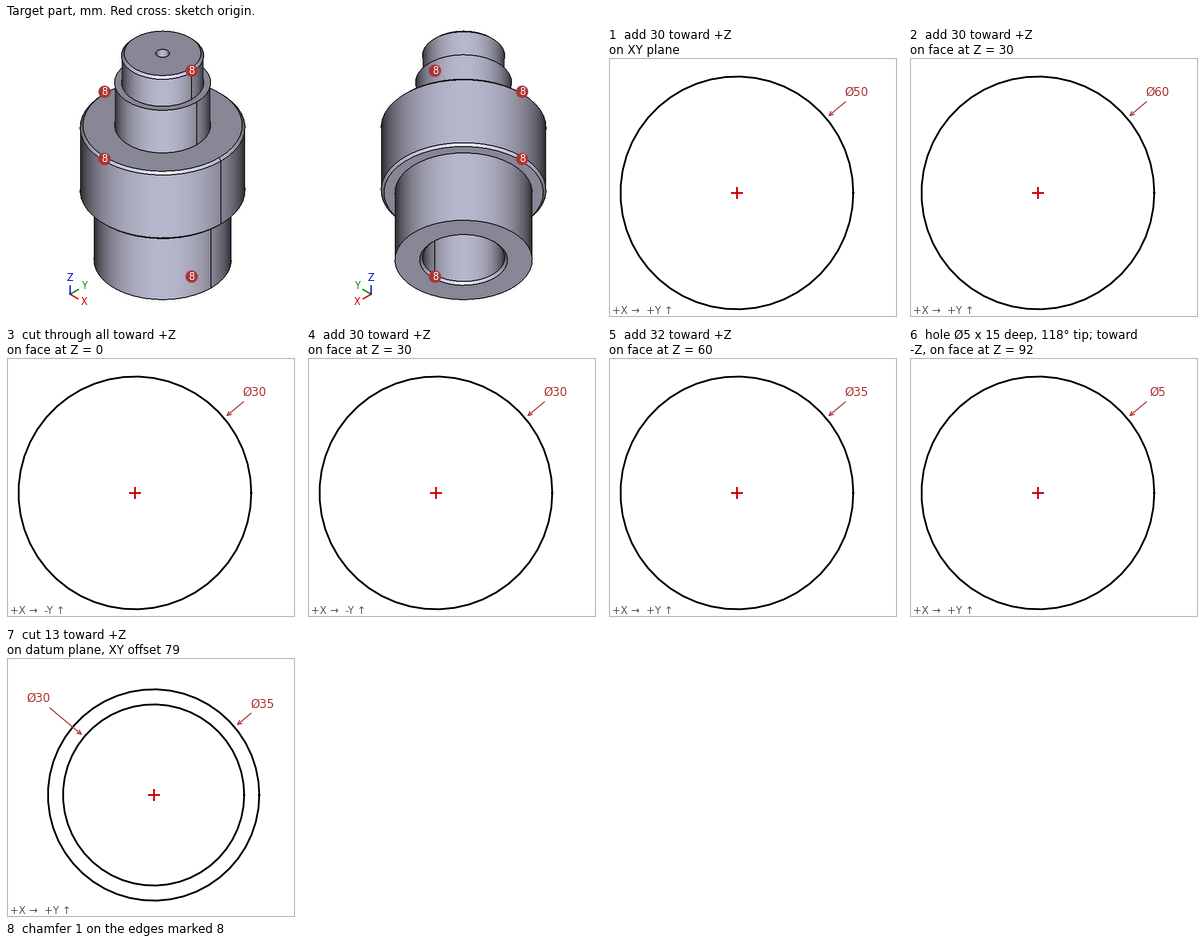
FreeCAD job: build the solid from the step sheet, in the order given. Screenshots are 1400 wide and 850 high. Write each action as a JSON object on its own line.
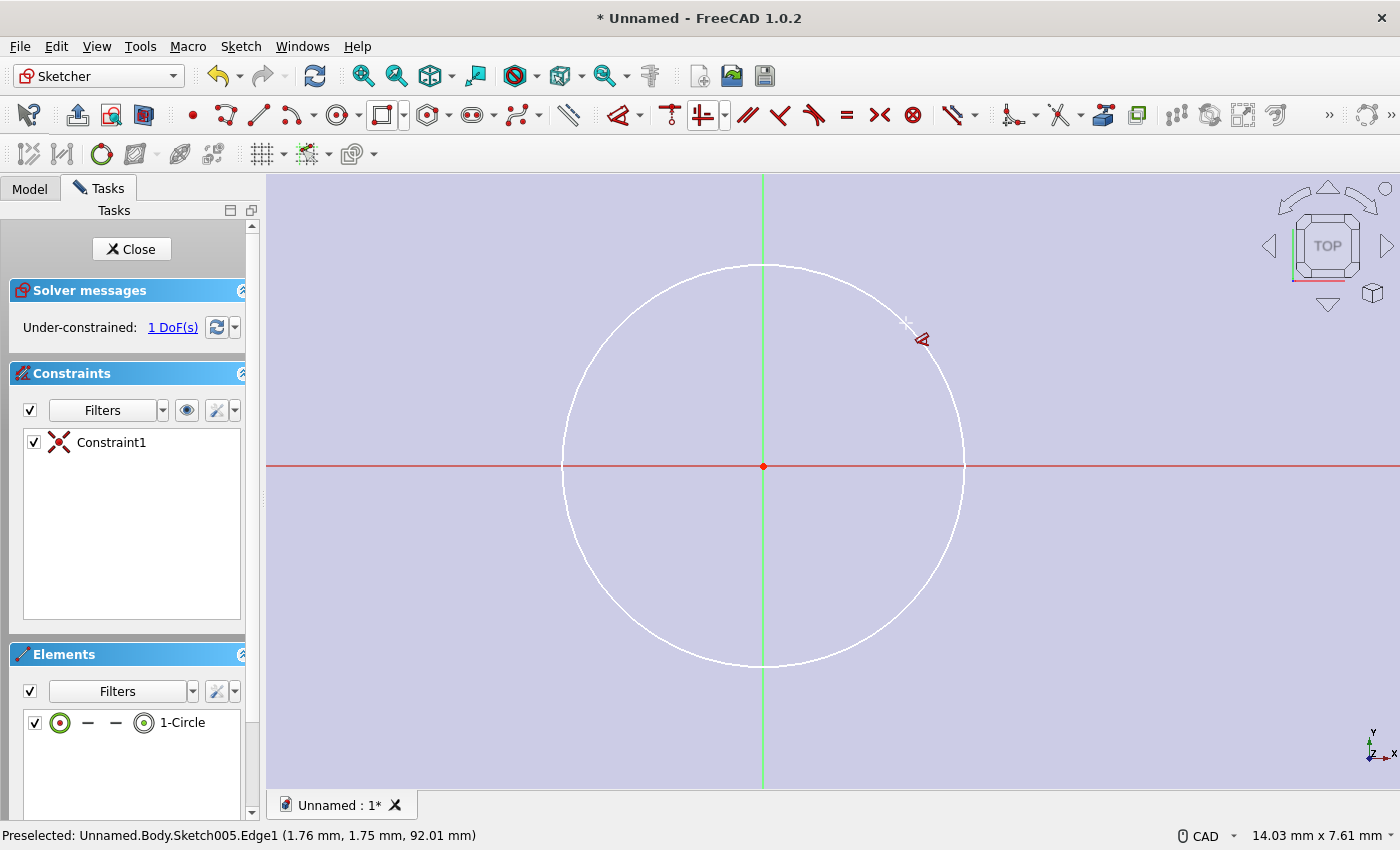
{"action": "left_click", "coordinate": [905, 323]}
{"action": "left_click", "coordinate": [928, 300]}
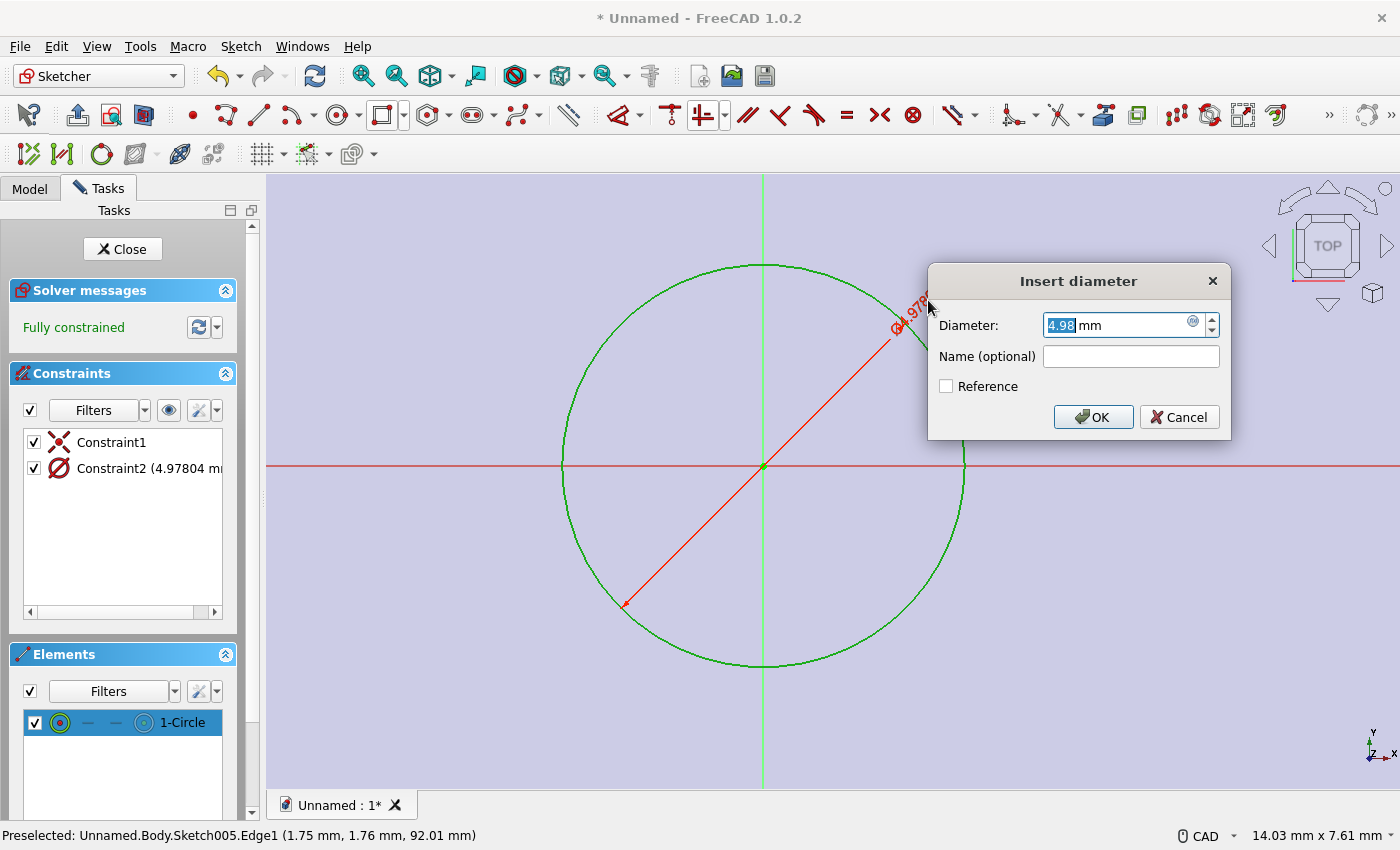
{"action": "type", "text": "5"}
{"action": "key", "text": "Return"}
{"action": "key", "text": "Escape"}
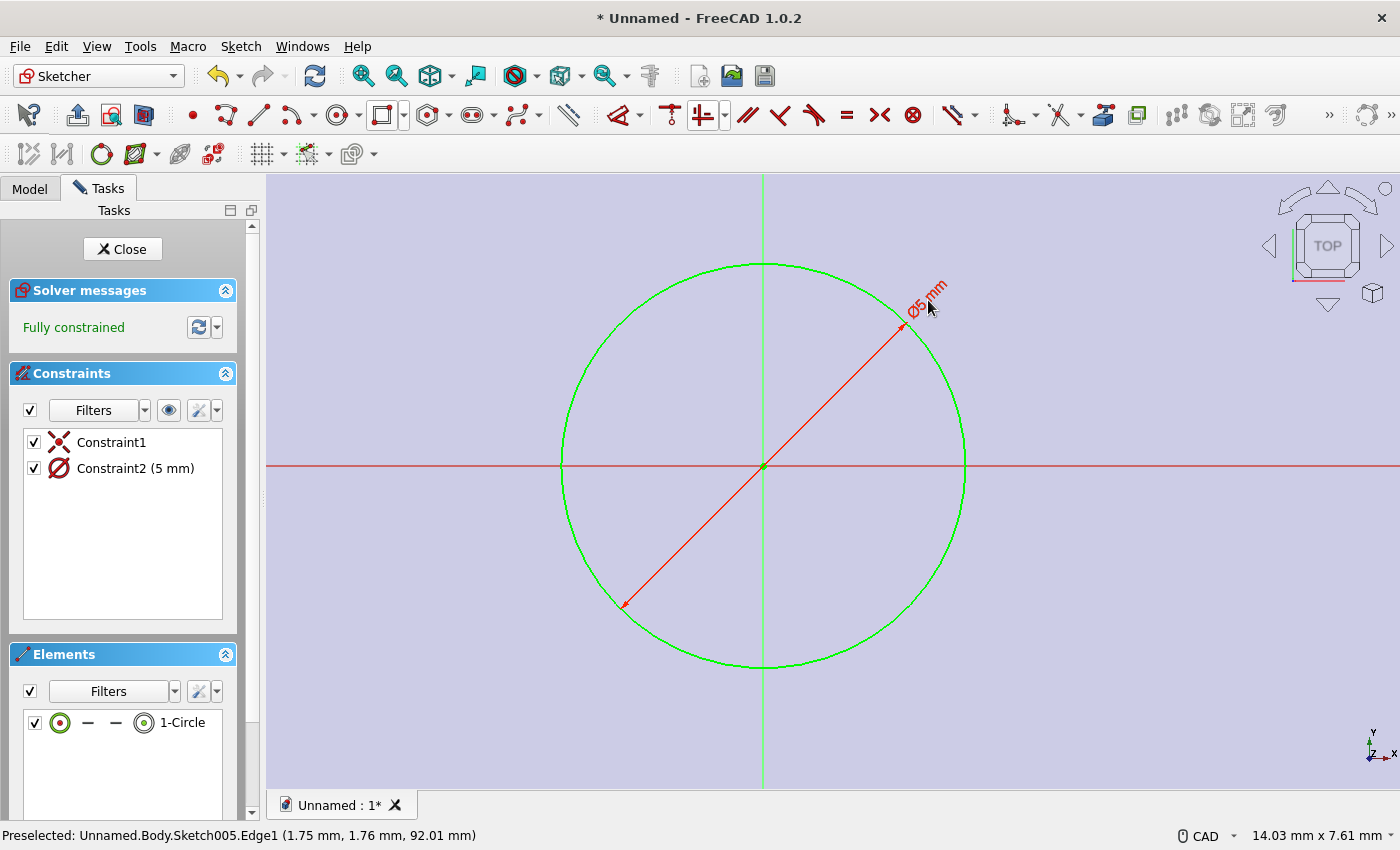
{"action": "left_click", "coordinate": [123, 249]}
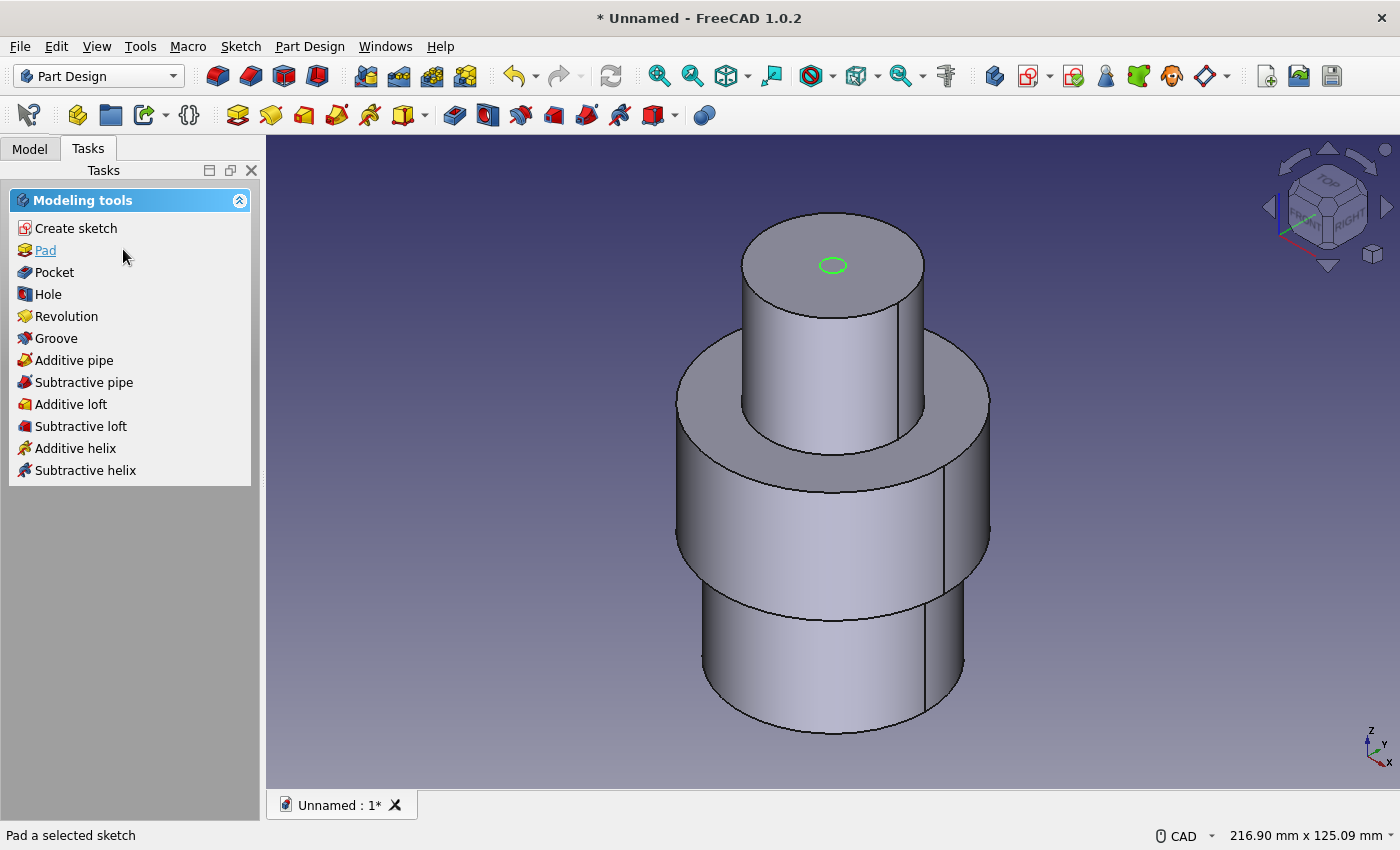
{"action": "left_click", "coordinate": [488, 116]}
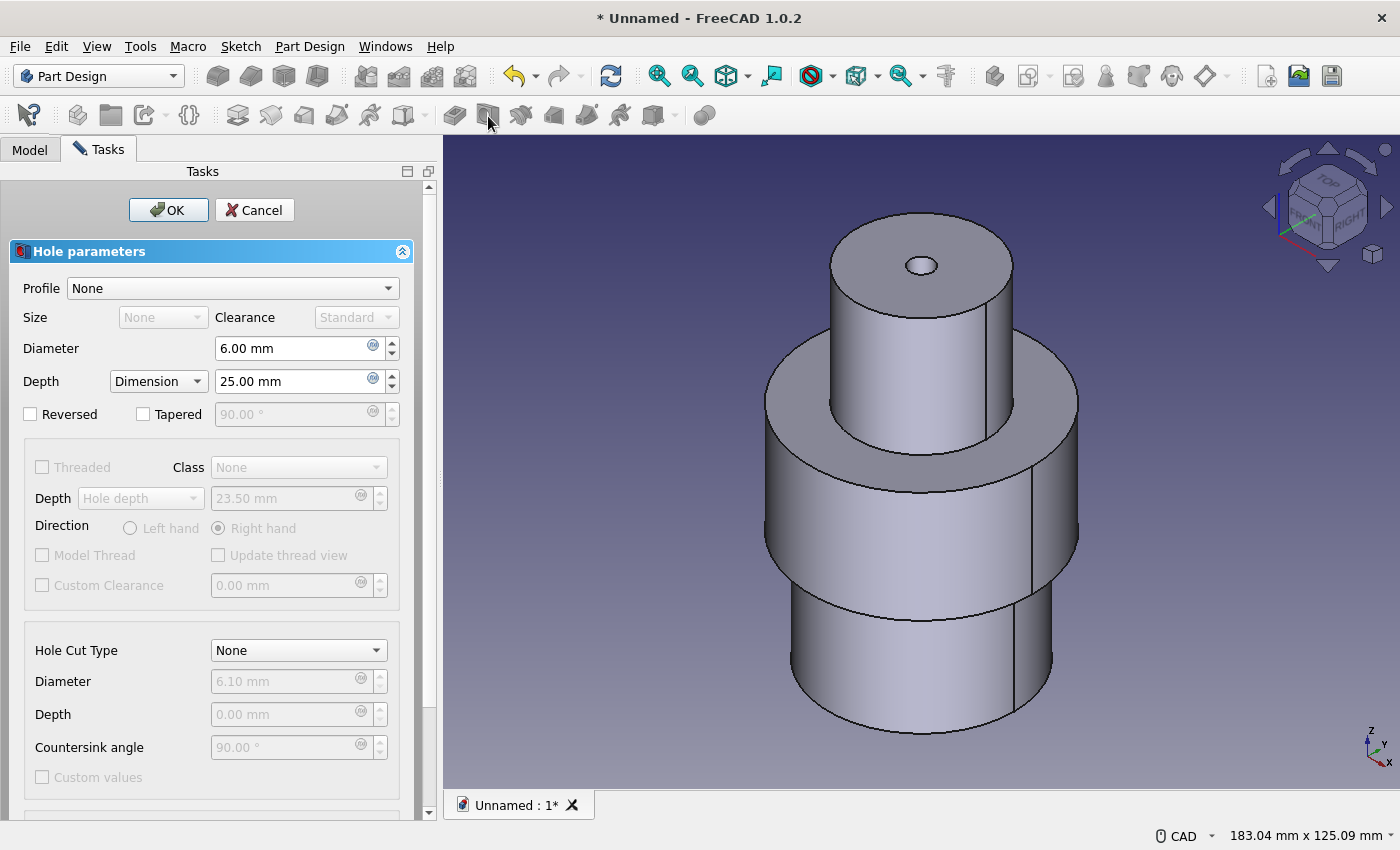
{"action": "triple_click", "coordinate": [300, 348]}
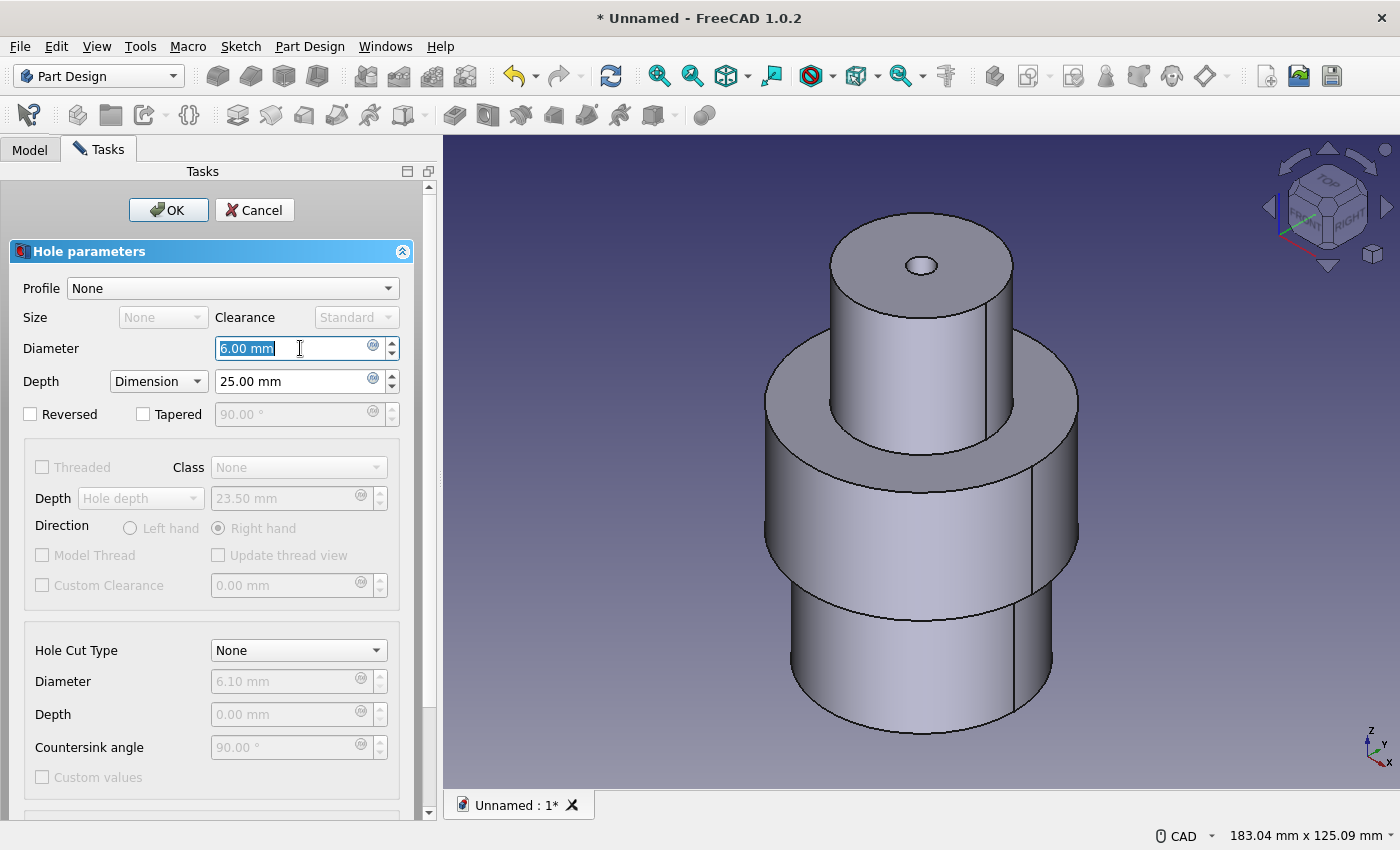
{"action": "type", "text": "5"}
{"action": "key", "text": "Tab"}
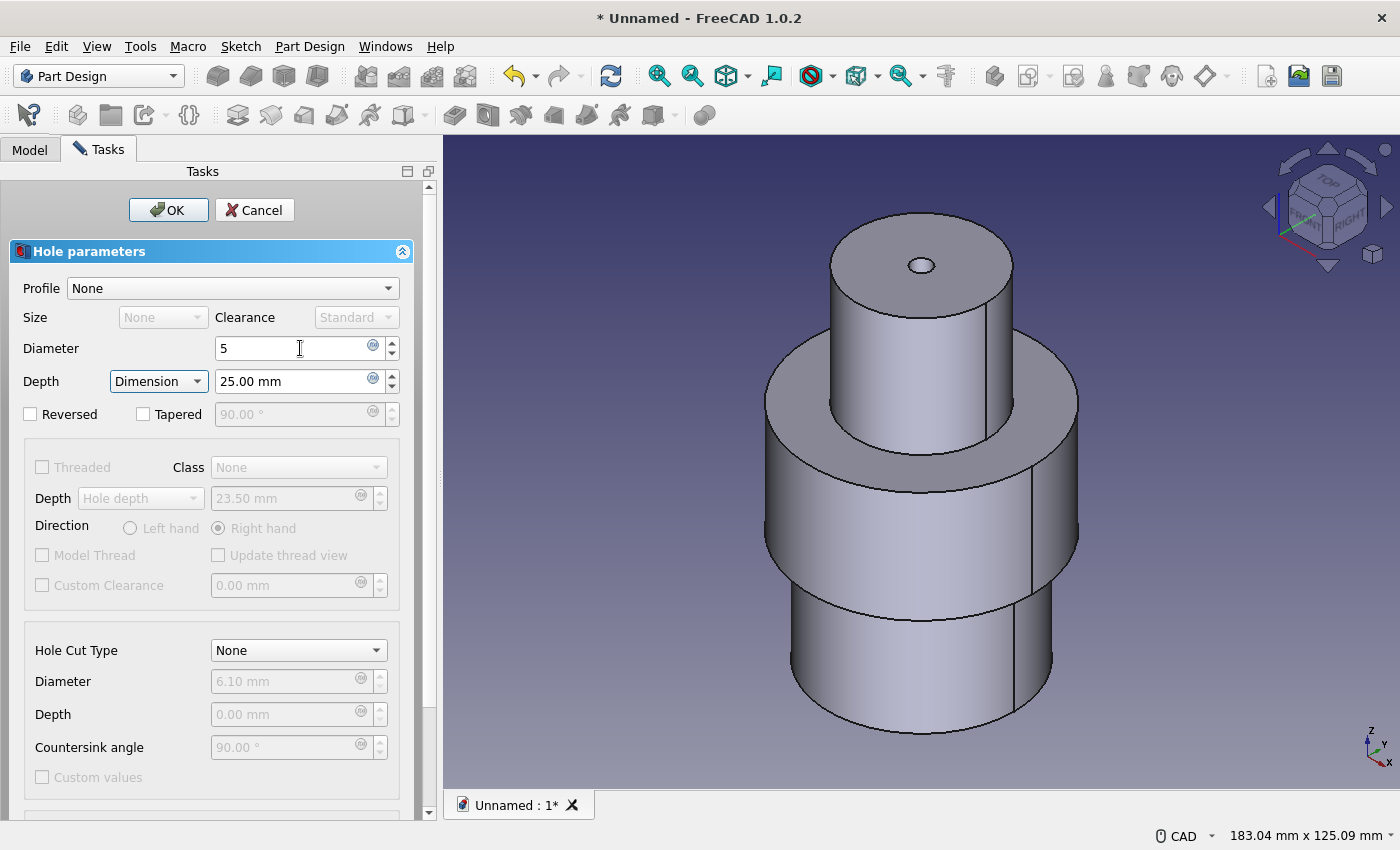
{"action": "triple_click", "coordinate": [300, 382]}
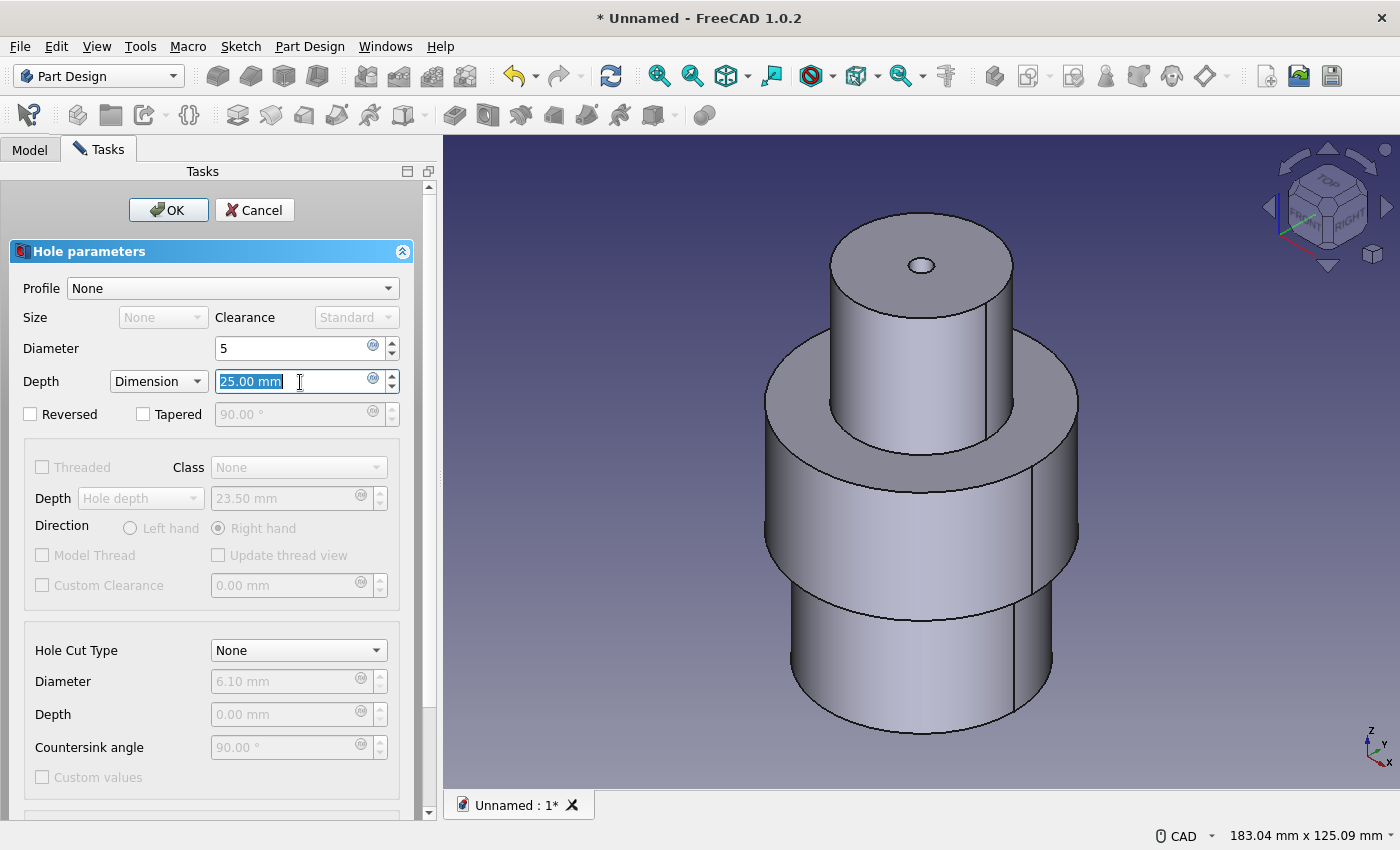
{"action": "type", "text": "15"}
{"action": "key", "text": "Tab"}